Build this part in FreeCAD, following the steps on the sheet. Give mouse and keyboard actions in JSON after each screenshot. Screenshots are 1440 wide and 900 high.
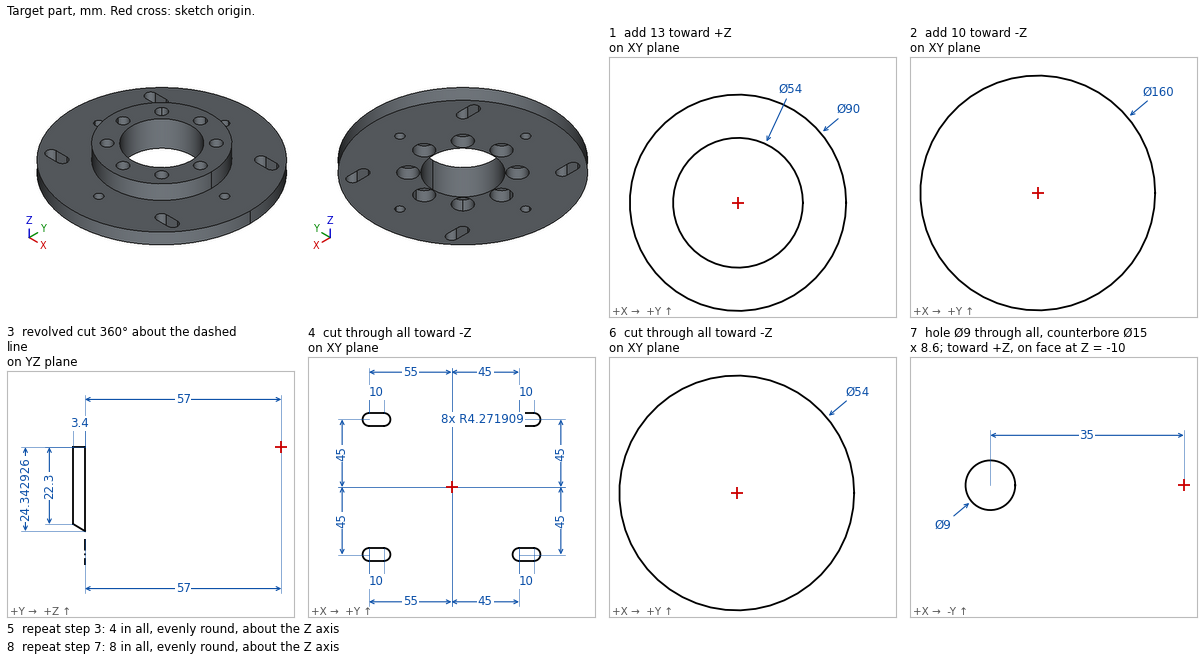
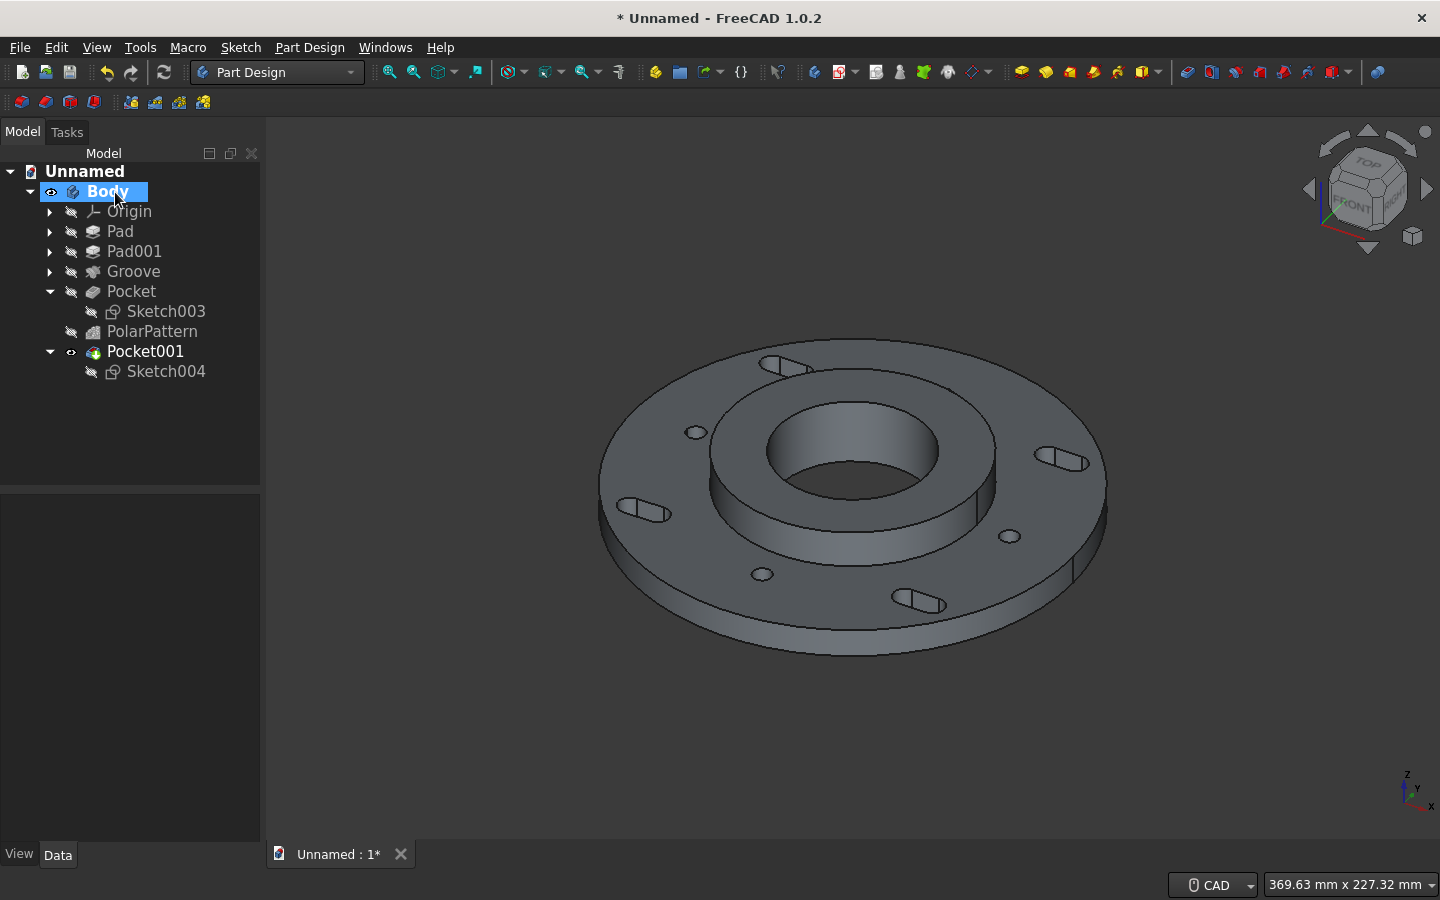
{"action": "key", "text": "5"}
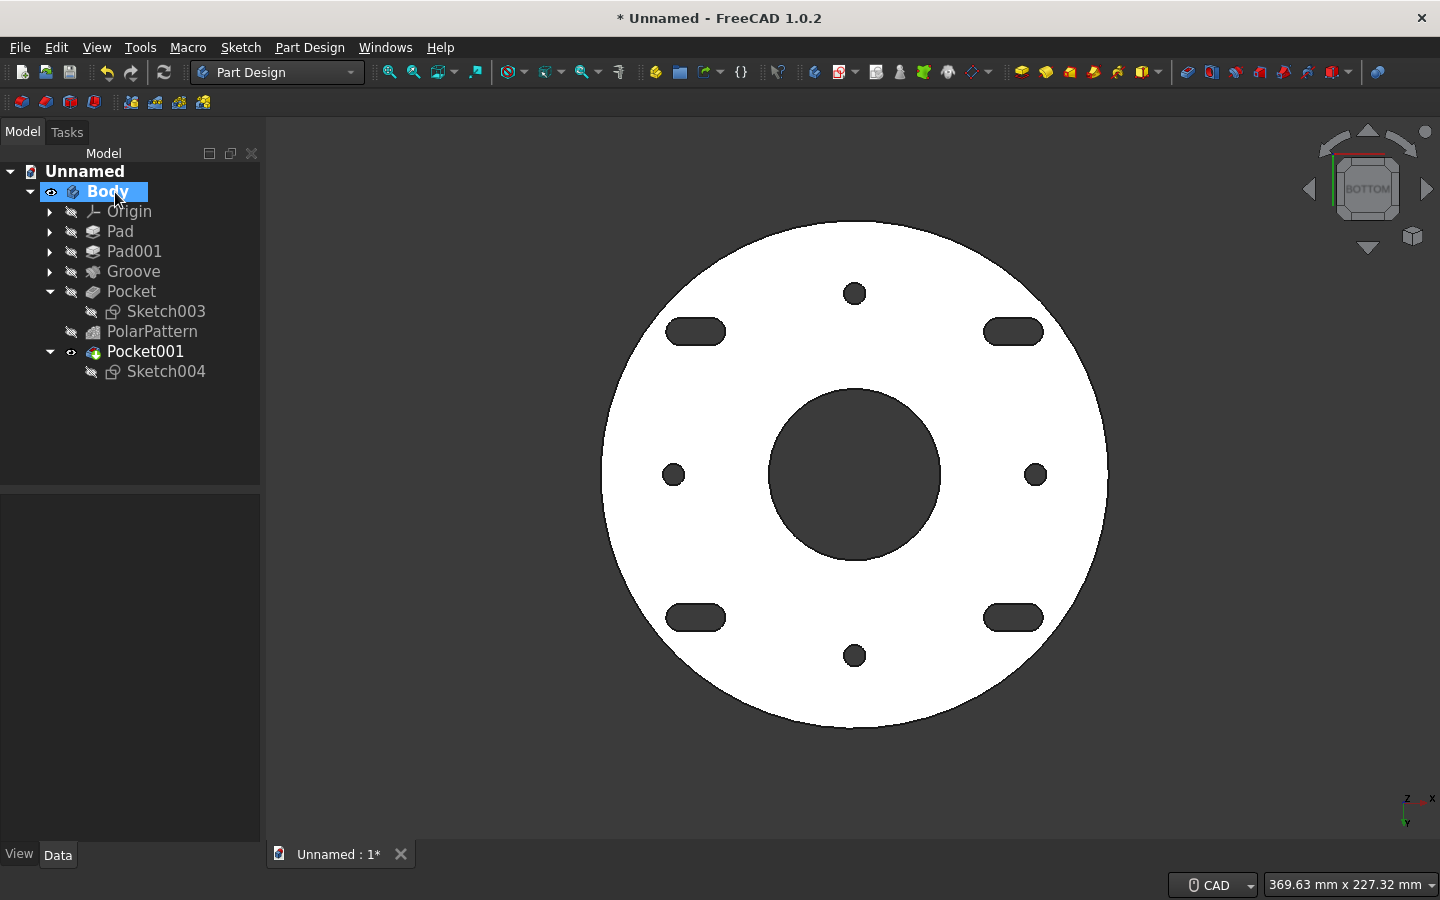
{"action": "left_click", "coordinate": [927, 619]}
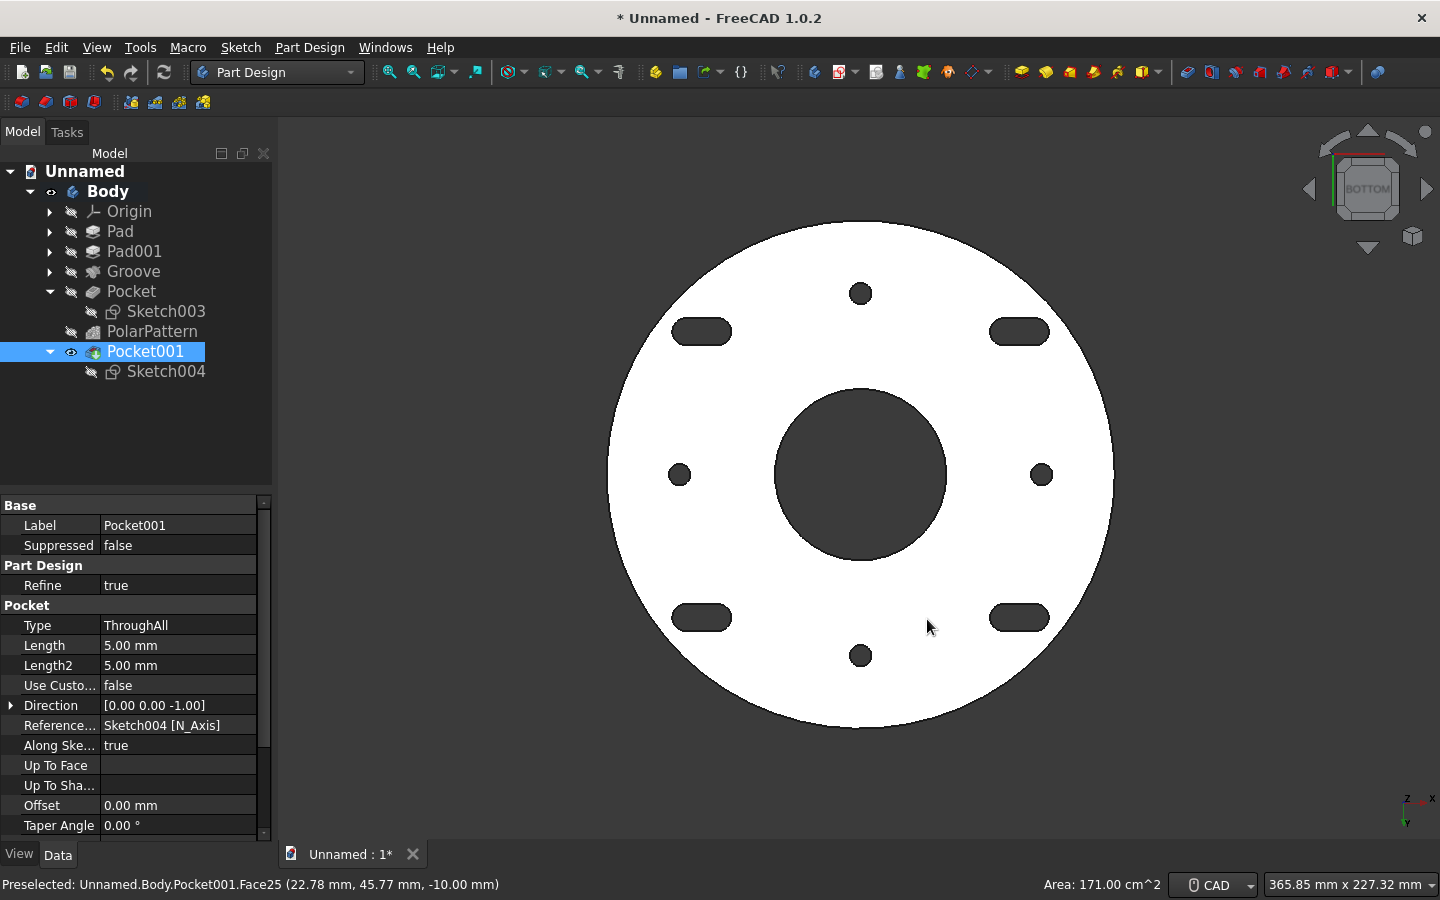
{"action": "left_click", "coordinate": [840, 72]}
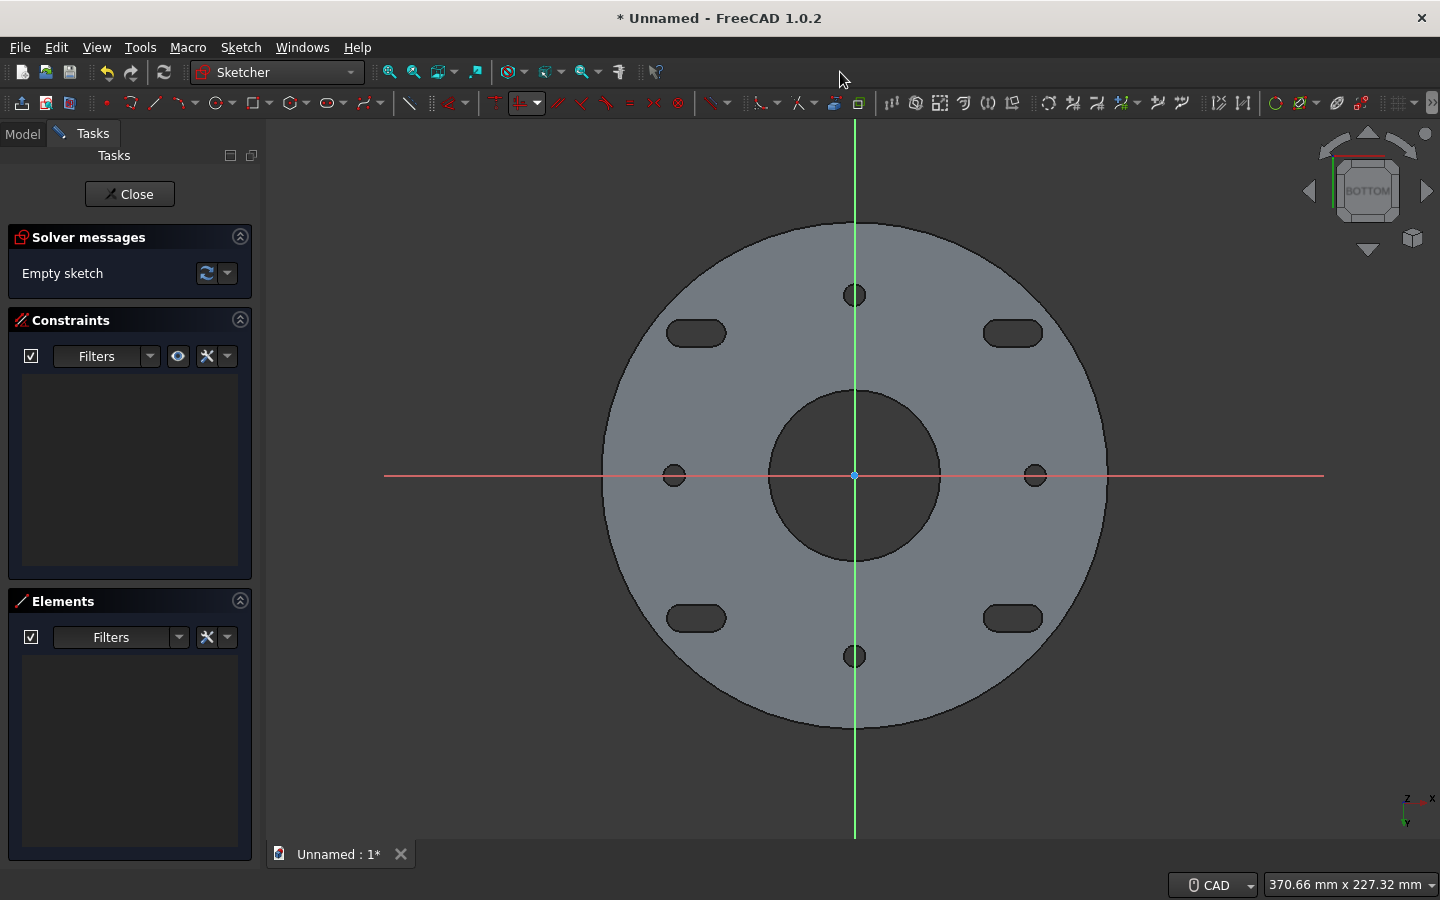
{"action": "scroll", "coordinate": [741, 475], "scroll_direction": "up", "scroll_amount": 14}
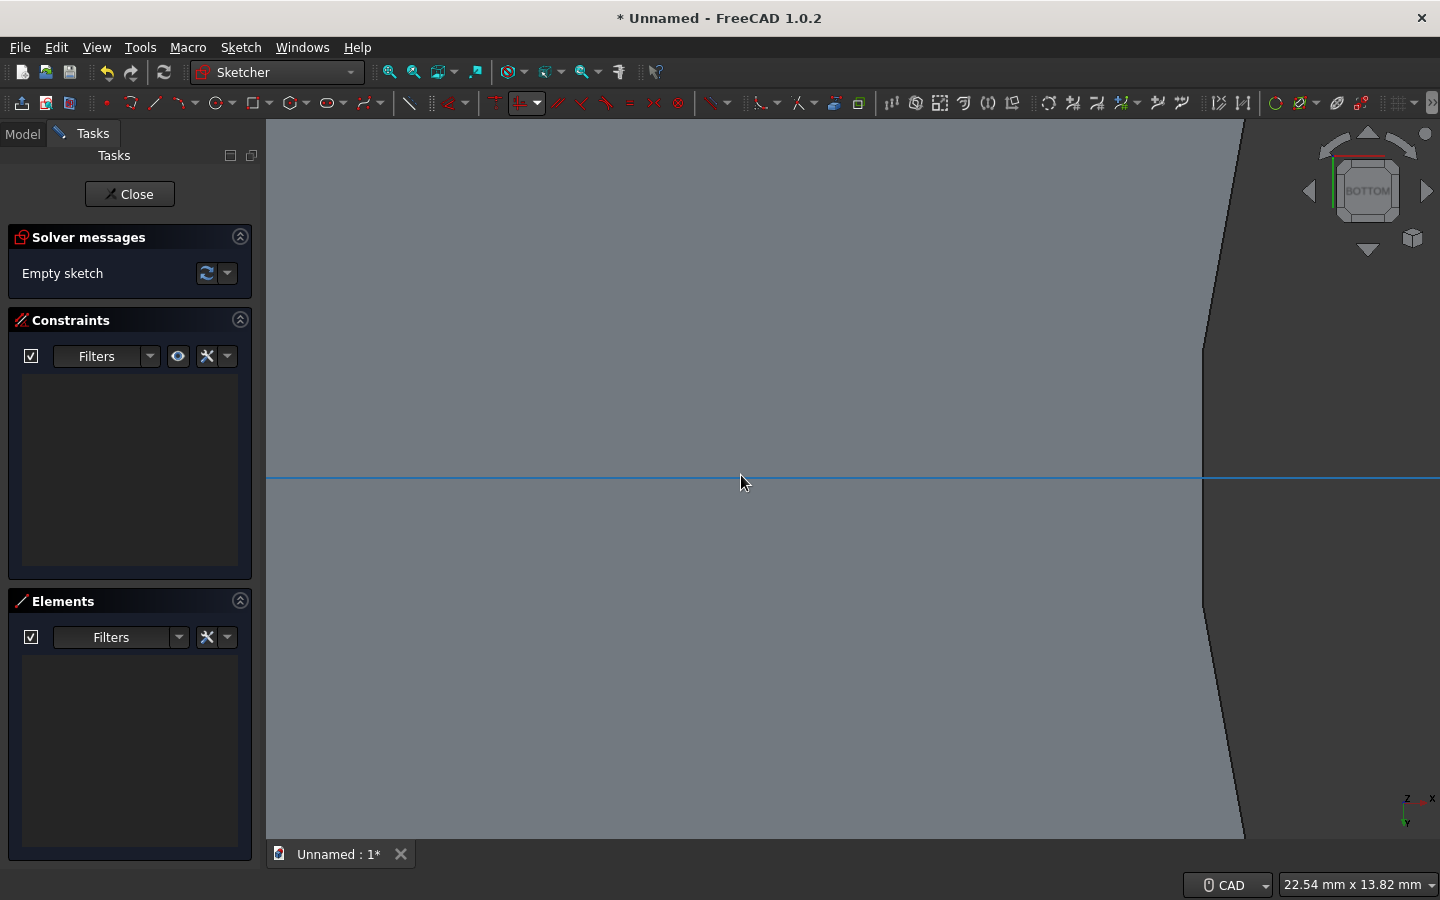
{"action": "key", "text": "g c"}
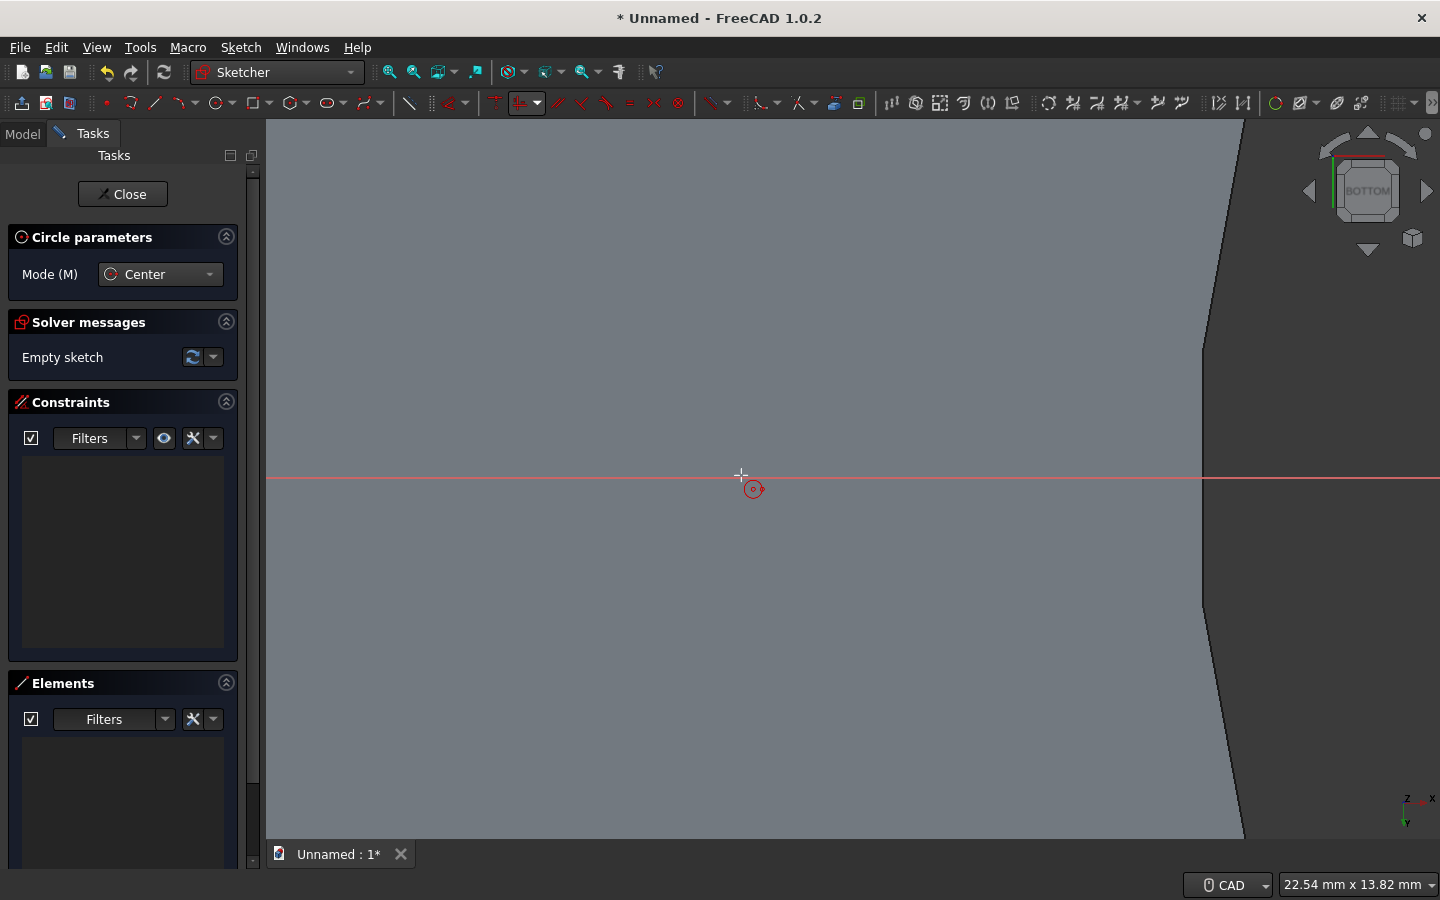
{"action": "left_click", "coordinate": [780, 478]}
{"action": "mouse_move", "coordinate": [946, 312]}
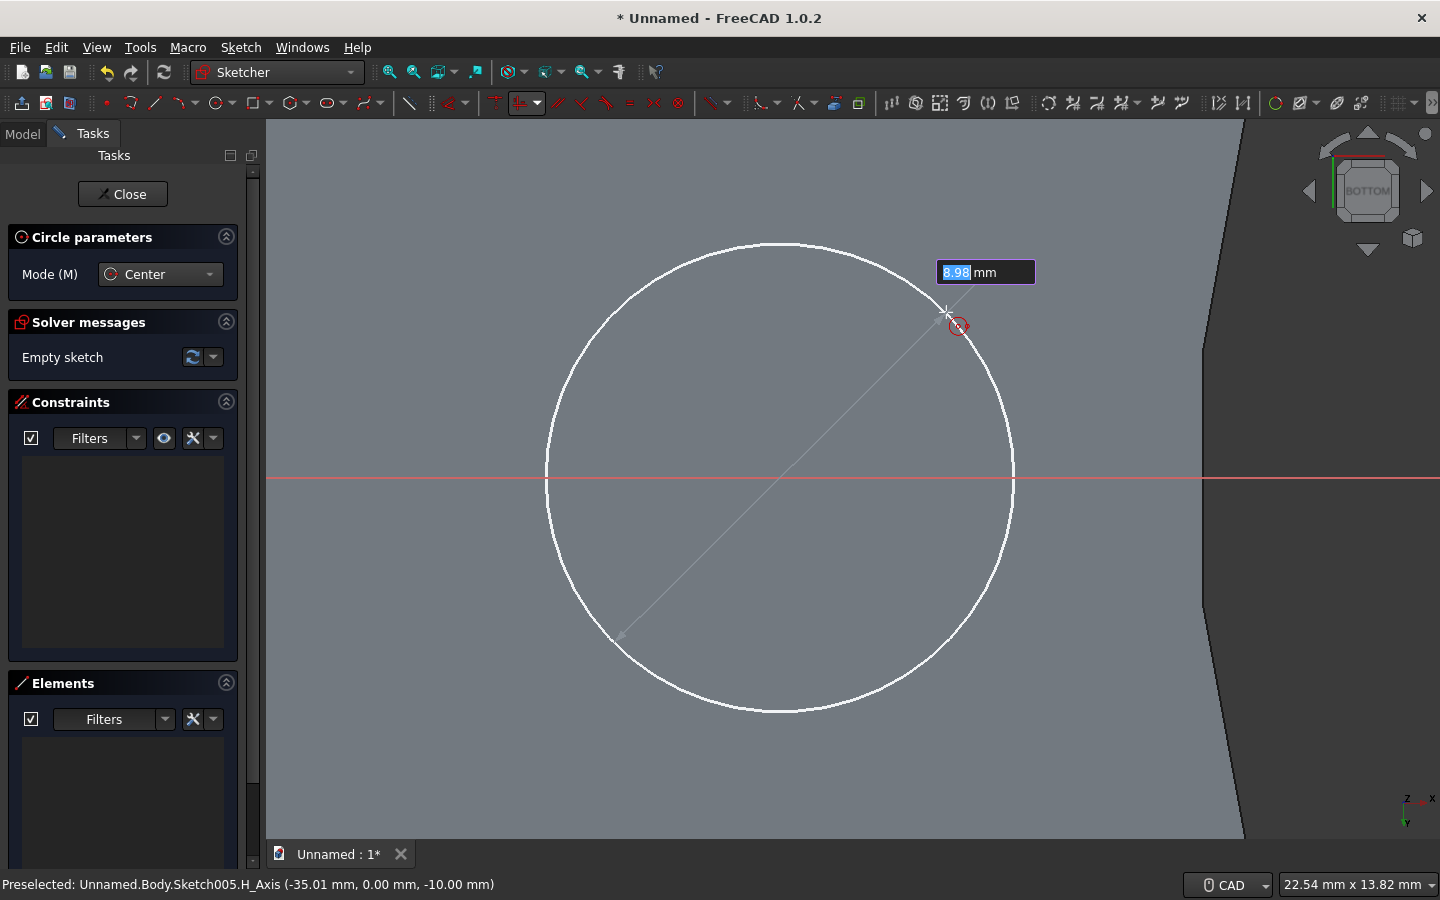
{"action": "type", "text": "9"}
{"action": "key", "text": "Return"}
{"action": "key", "text": "Escape"}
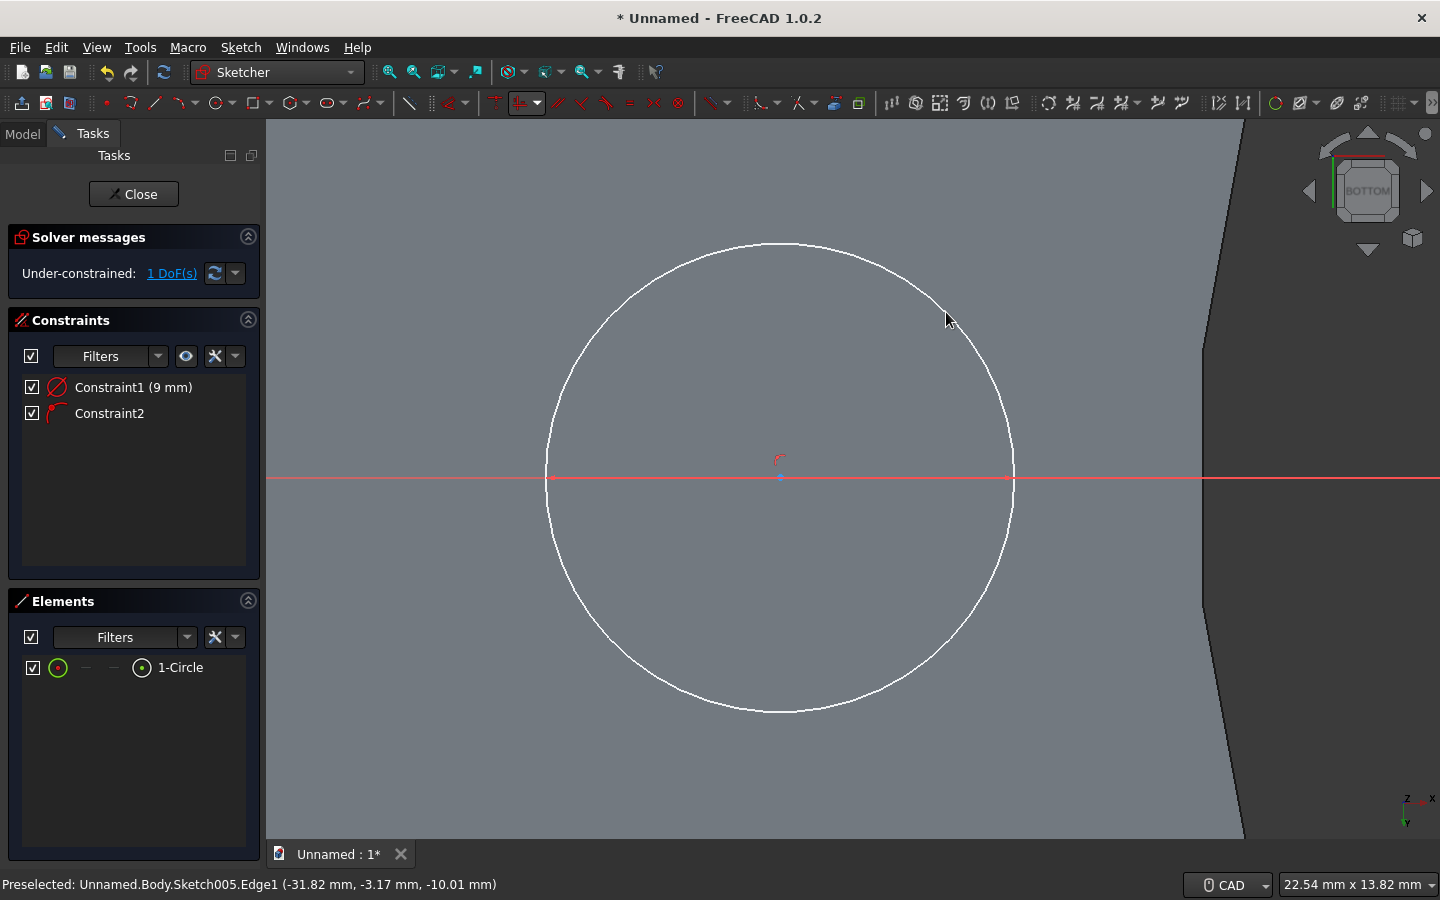
{"action": "key", "text": "d"}